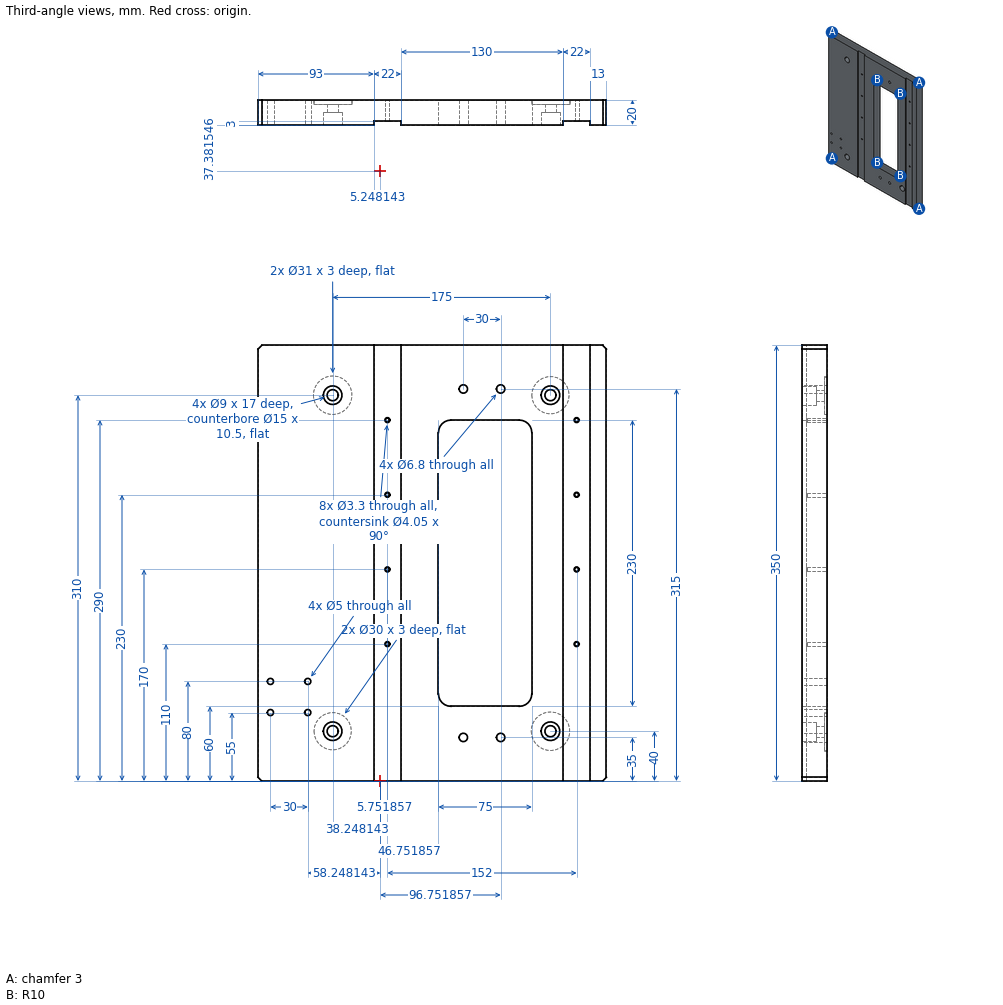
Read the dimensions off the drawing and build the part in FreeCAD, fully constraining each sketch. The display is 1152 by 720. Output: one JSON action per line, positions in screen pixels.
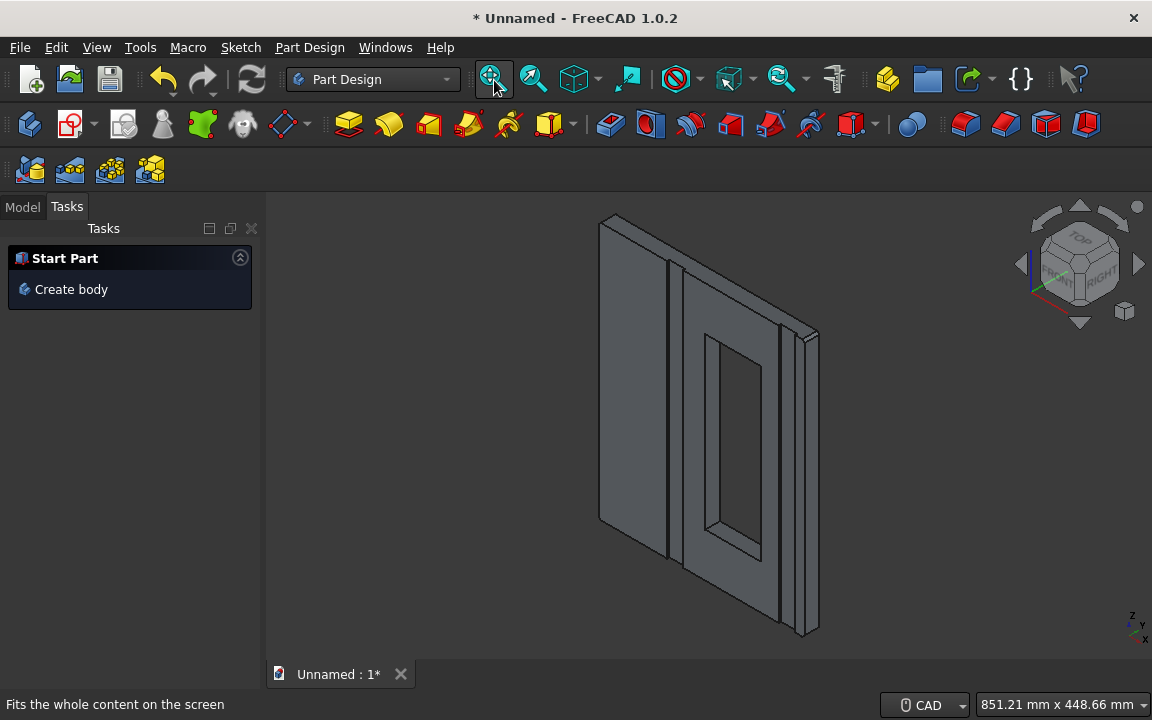
{"action": "key", "text": "2"}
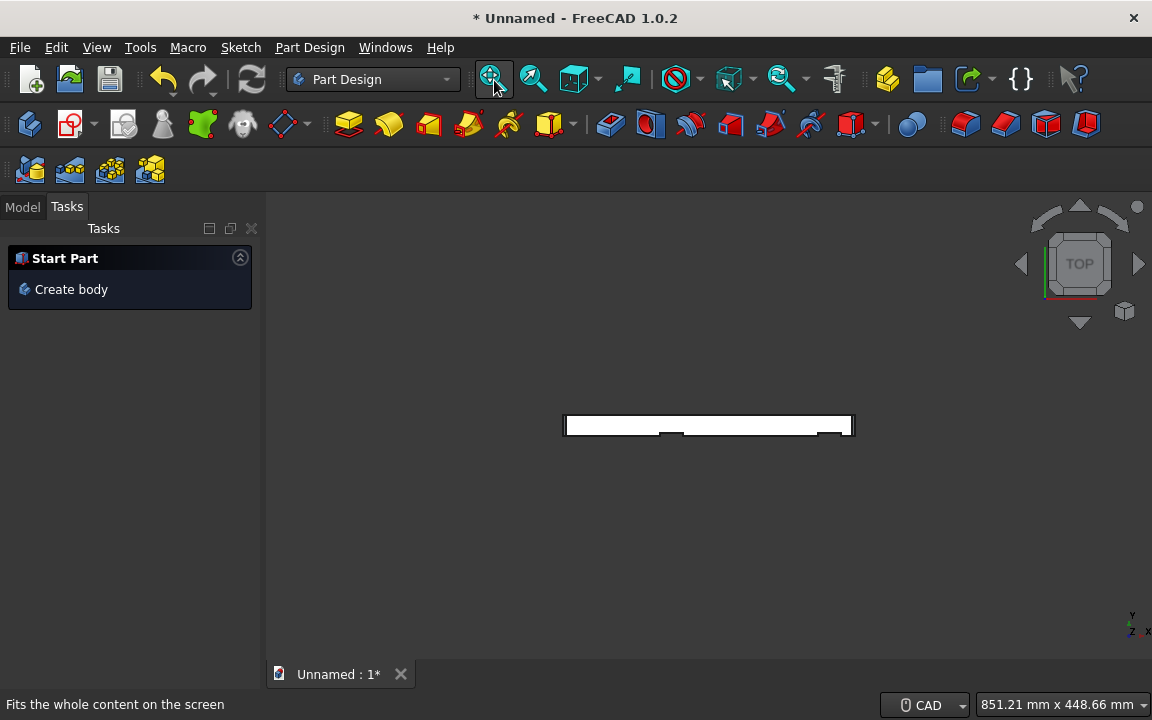
{"action": "left_click", "coordinate": [494, 80]}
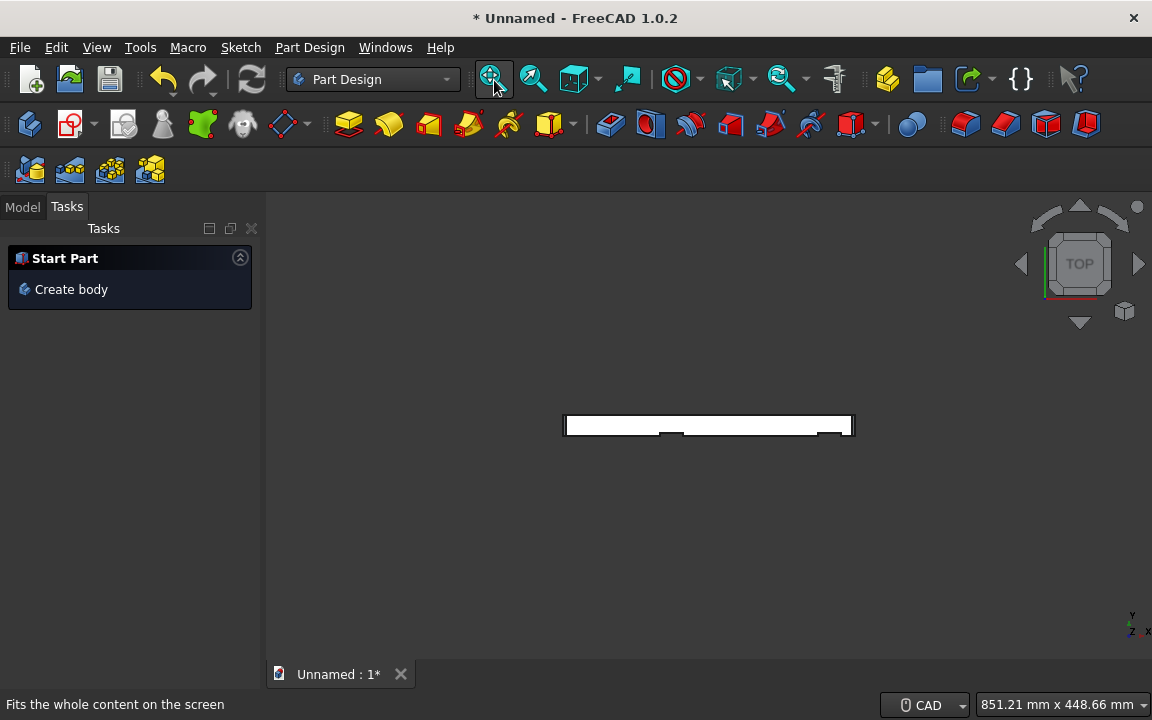
{"action": "scroll", "coordinate": [714, 424], "scroll_direction": "up", "scroll_amount": 4}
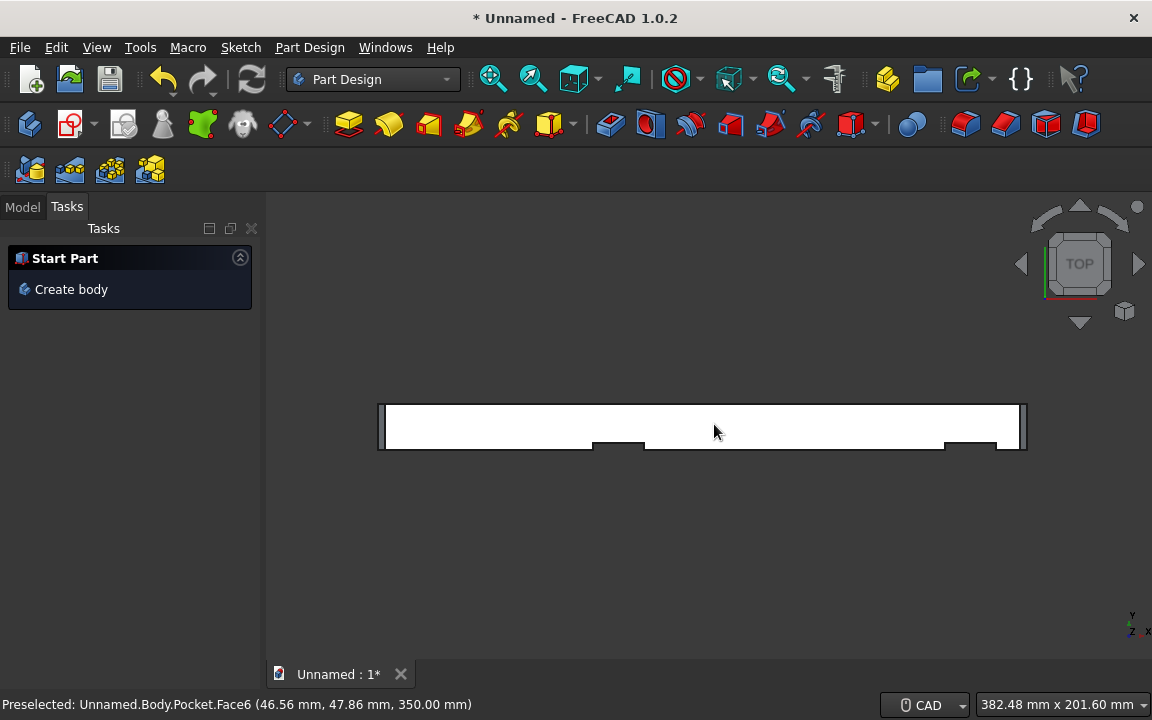
{"action": "left_click", "coordinate": [494, 80]}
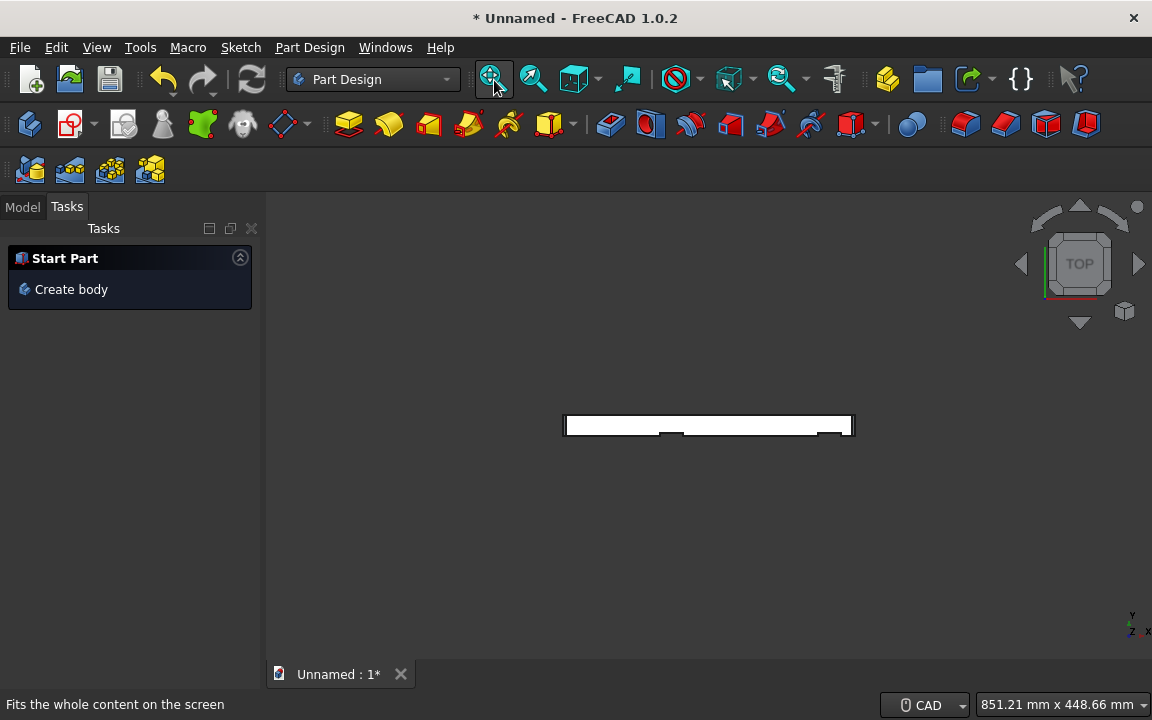
{"action": "key", "text": "0"}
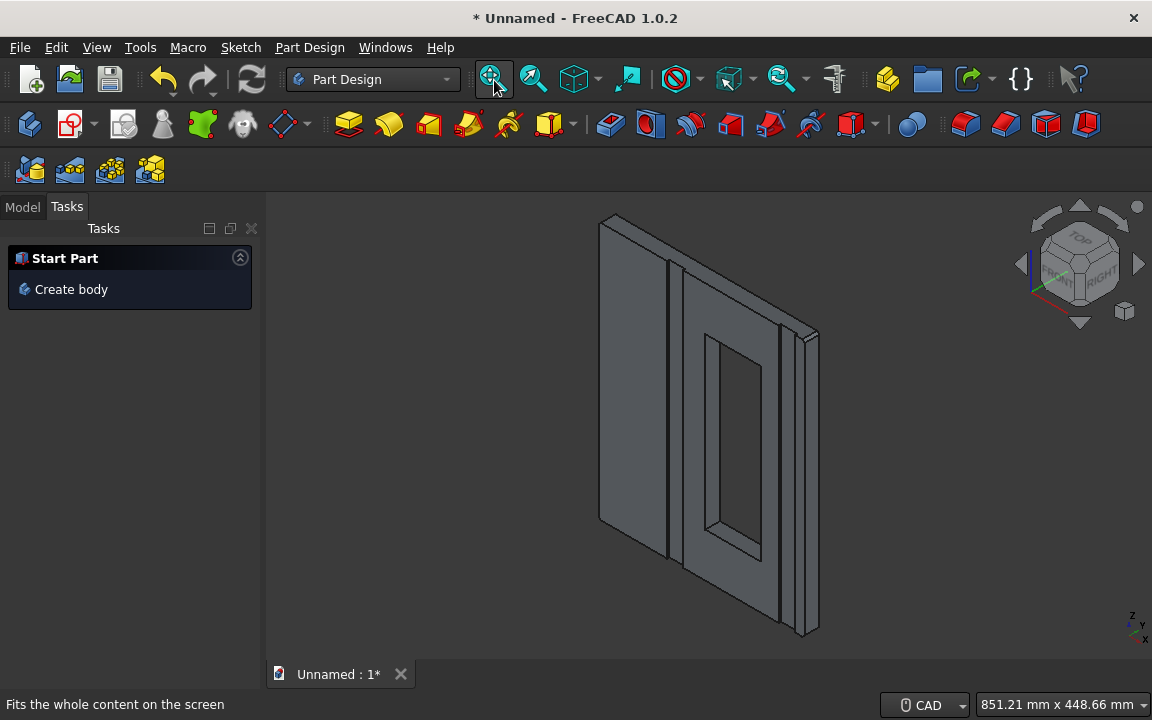
{"action": "scroll", "coordinate": [713, 524], "scroll_direction": "up", "scroll_amount": 4}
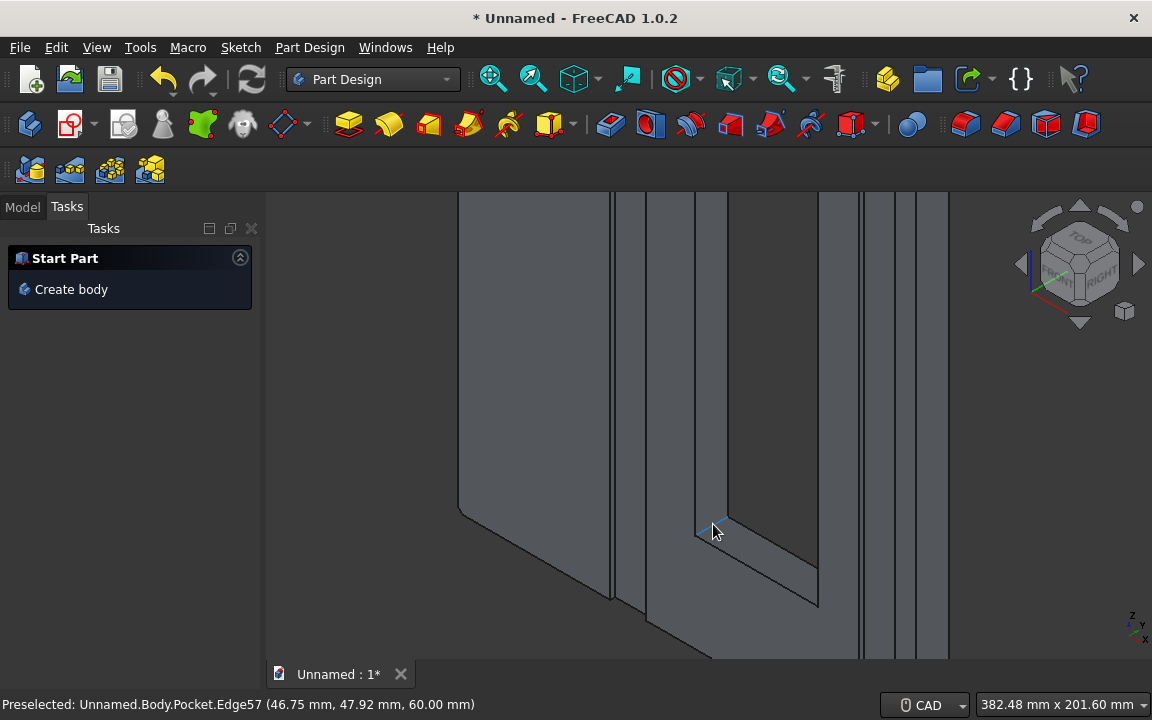
{"action": "left_click", "coordinate": [494, 80]}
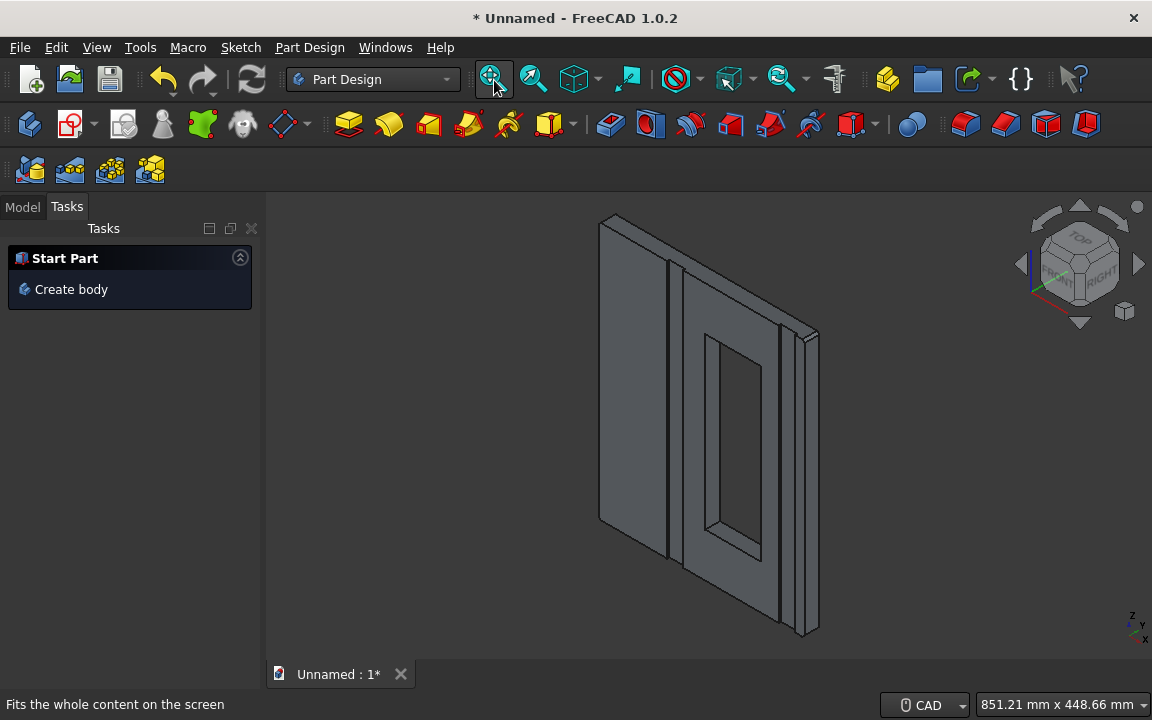
{"action": "key", "text": "1"}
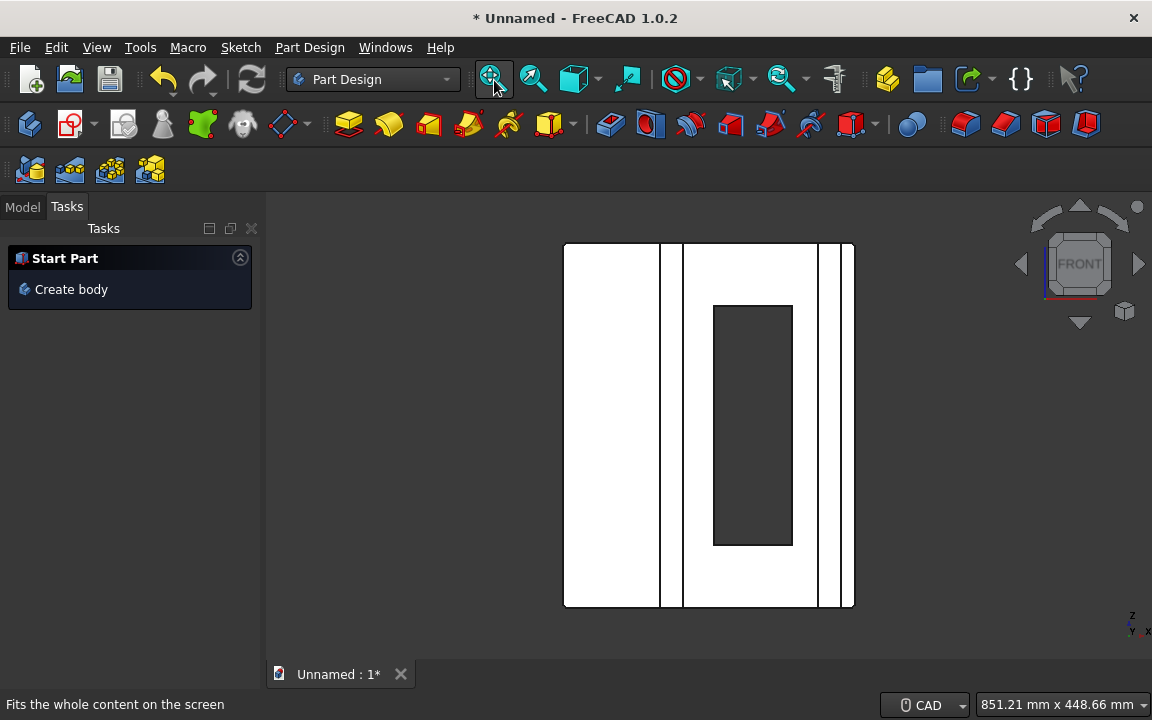
{"action": "scroll", "coordinate": [714, 544], "scroll_direction": "up", "scroll_amount": 4}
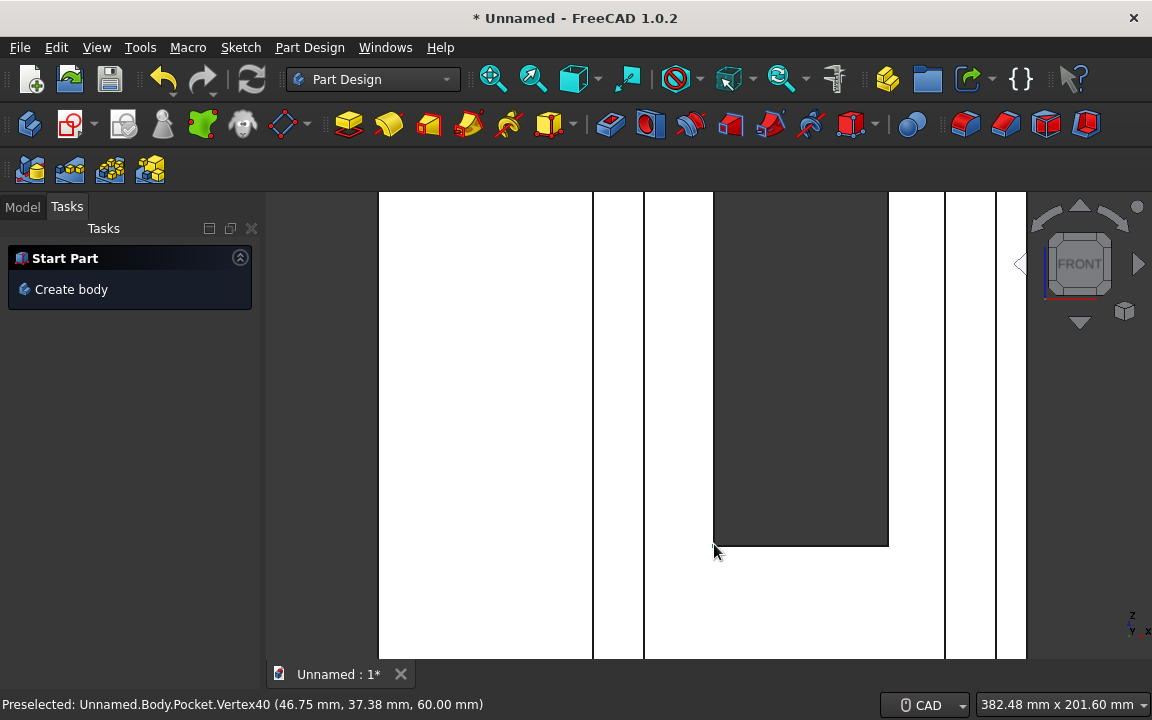
{"action": "left_click", "coordinate": [494, 80]}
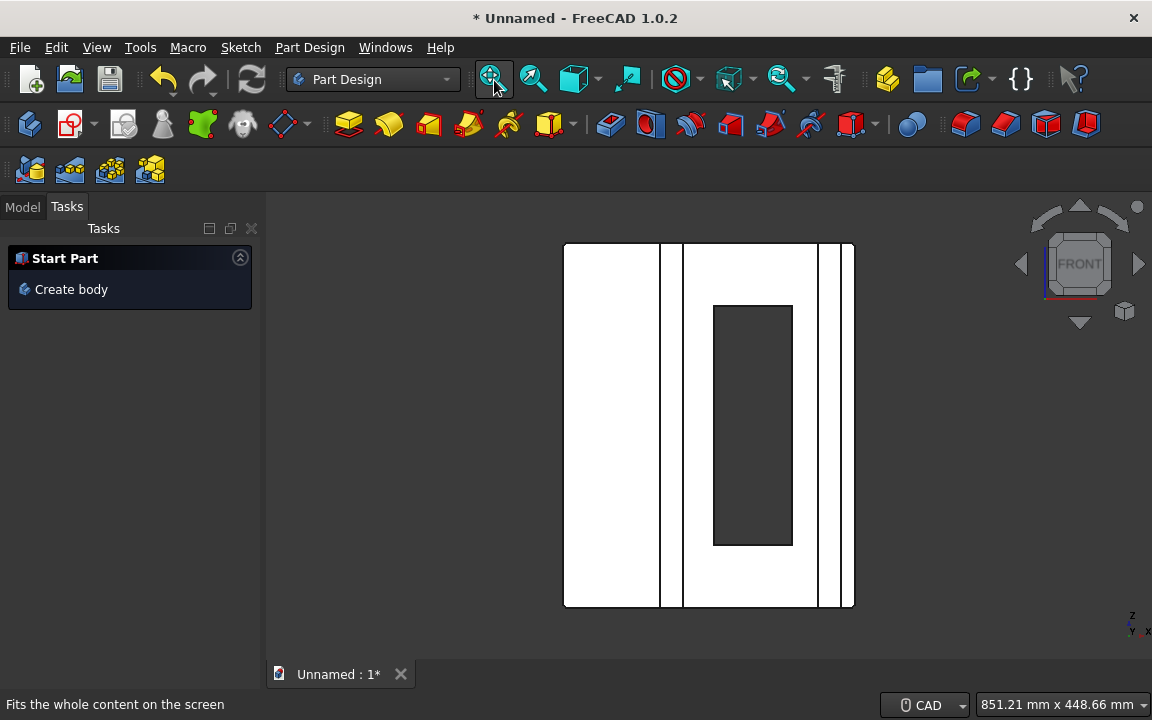
{"action": "key", "text": "3"}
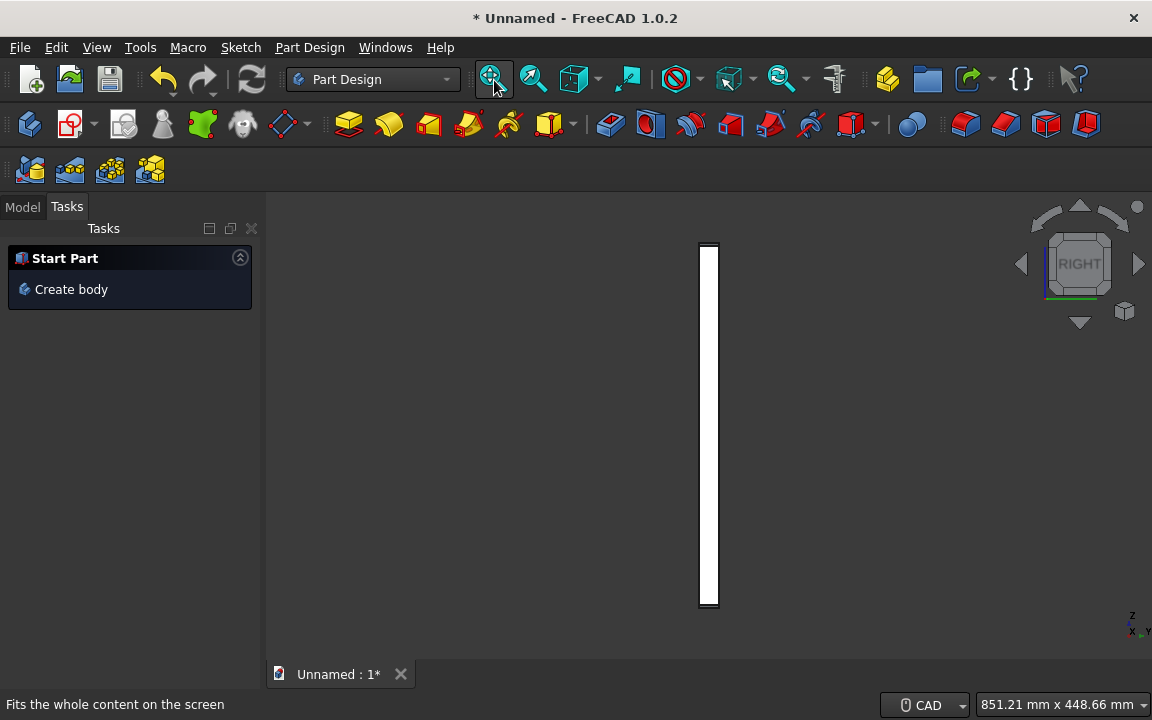
{"action": "scroll", "coordinate": [709, 544], "scroll_direction": "up", "scroll_amount": 4}